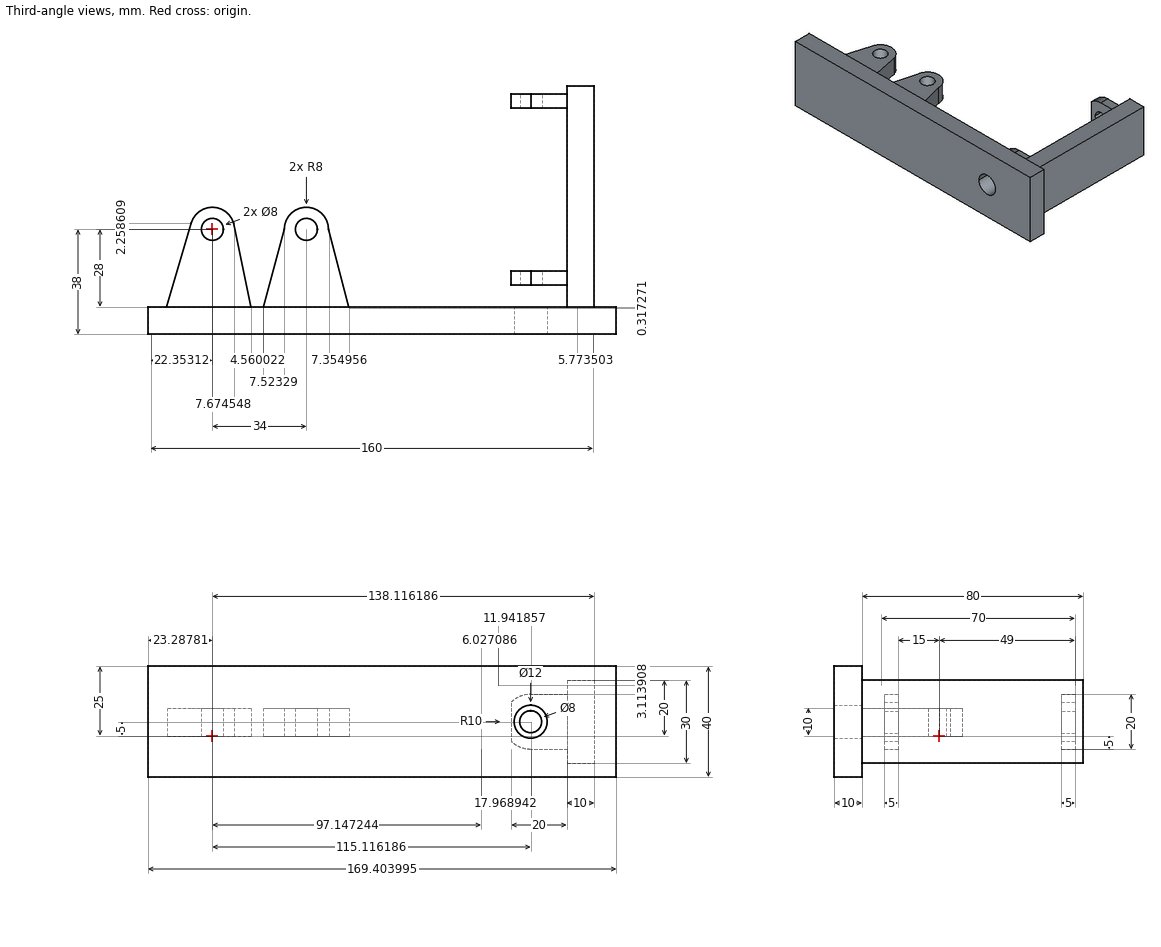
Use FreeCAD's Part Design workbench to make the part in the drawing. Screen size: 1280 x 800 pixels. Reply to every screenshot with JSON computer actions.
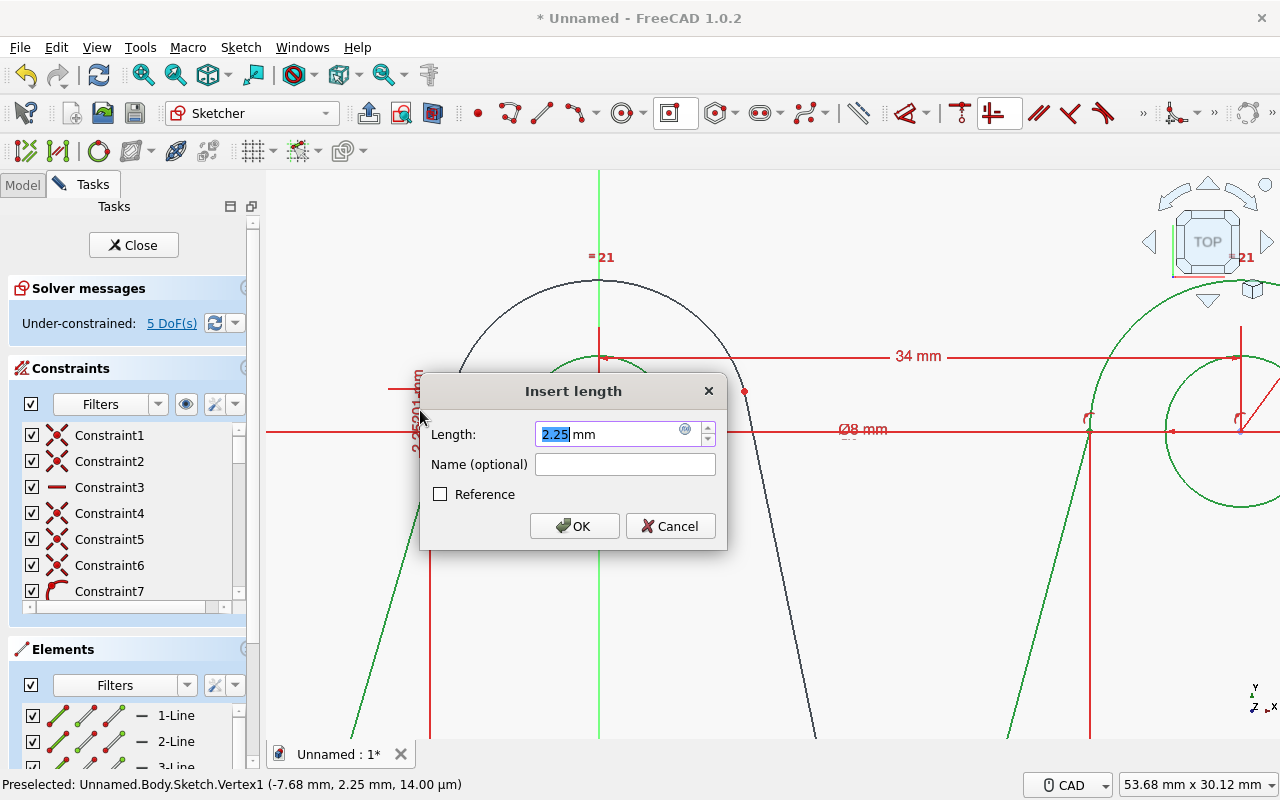
{"action": "type", "text": "2.258609"}
{"action": "key", "text": "Return"}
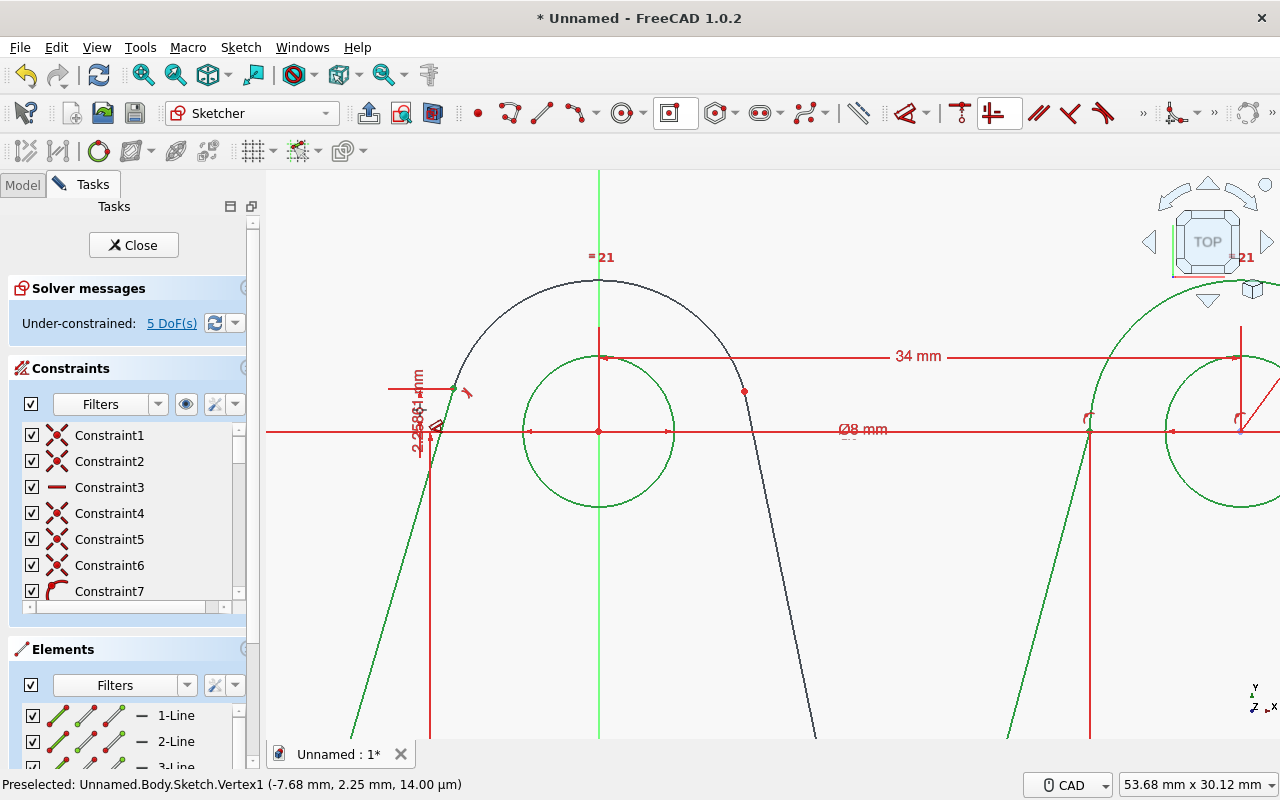
{"action": "scroll", "coordinate": [456, 389], "scroll_direction": "down", "scroll_amount": 8}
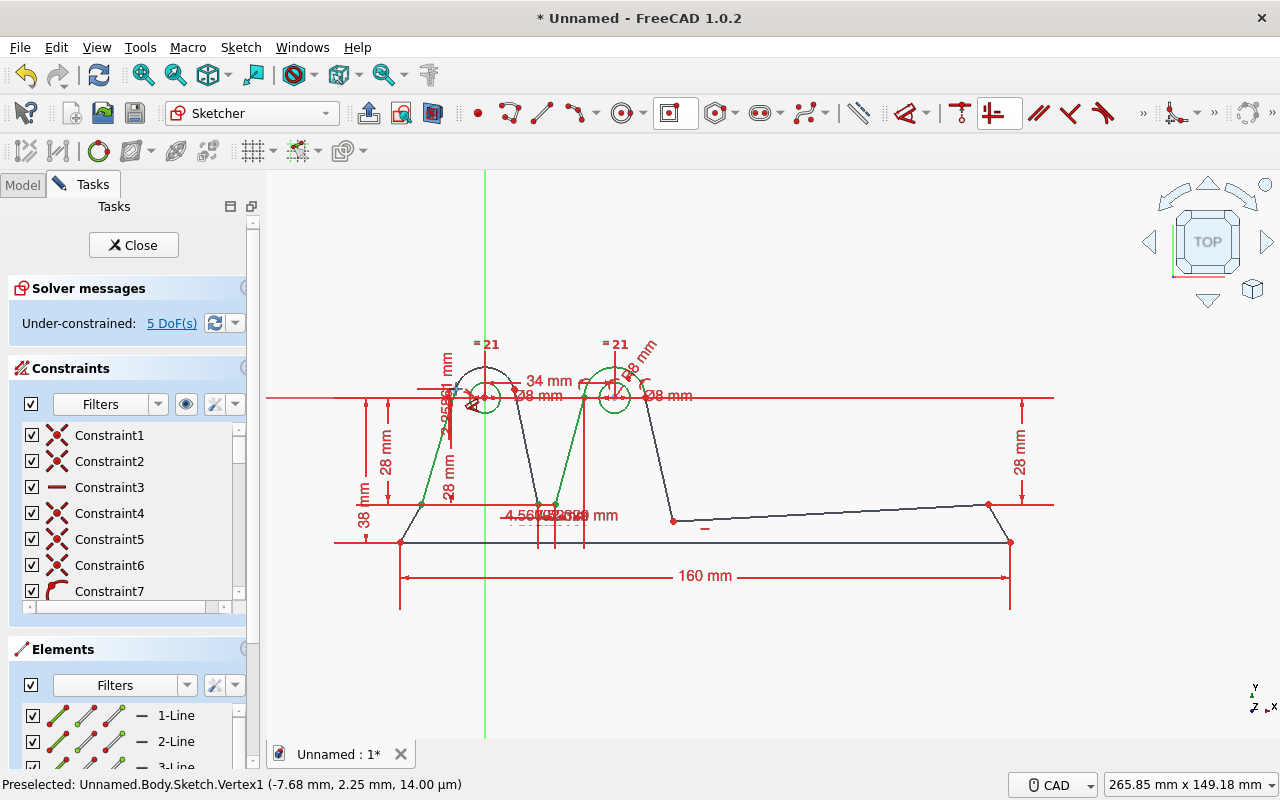
{"action": "left_click", "coordinate": [400, 543]}
{"action": "left_click", "coordinate": [442, 577]}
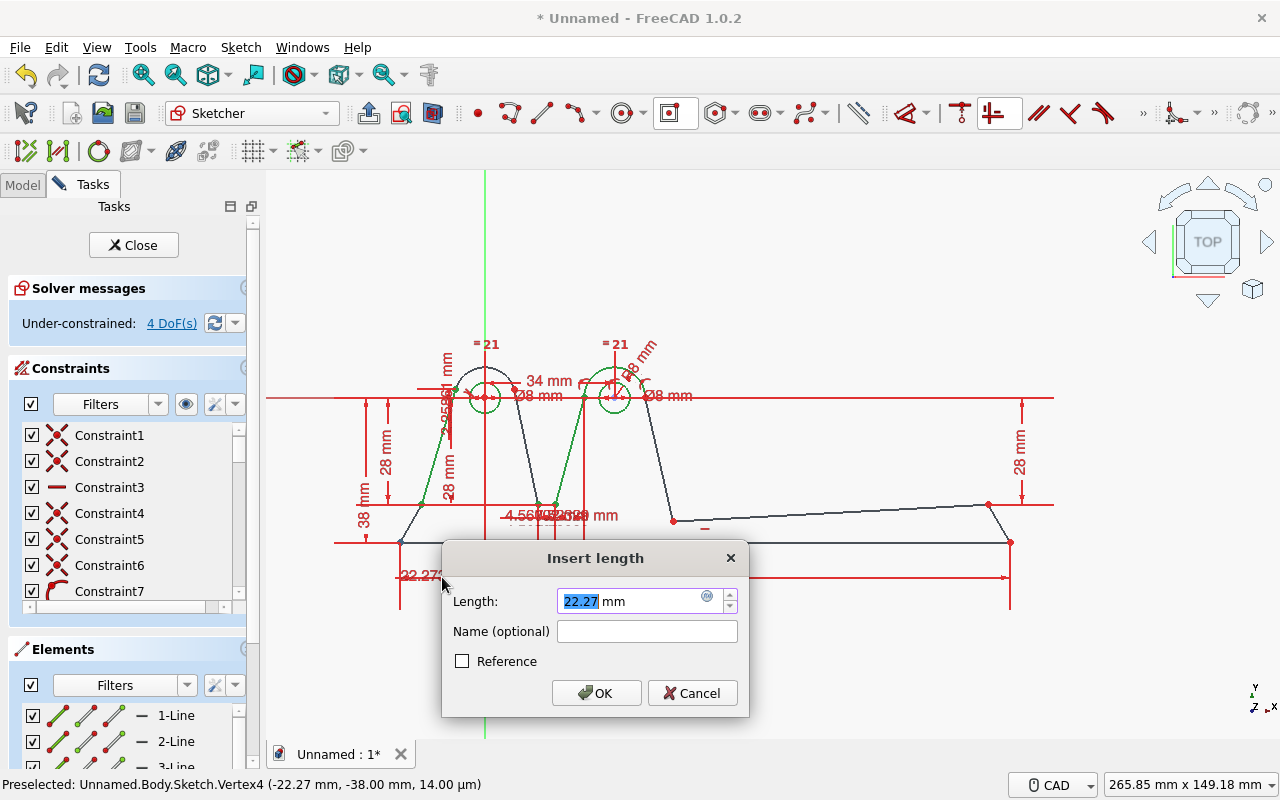
{"action": "type", "text": "22.35312"}
{"action": "key", "text": "Return"}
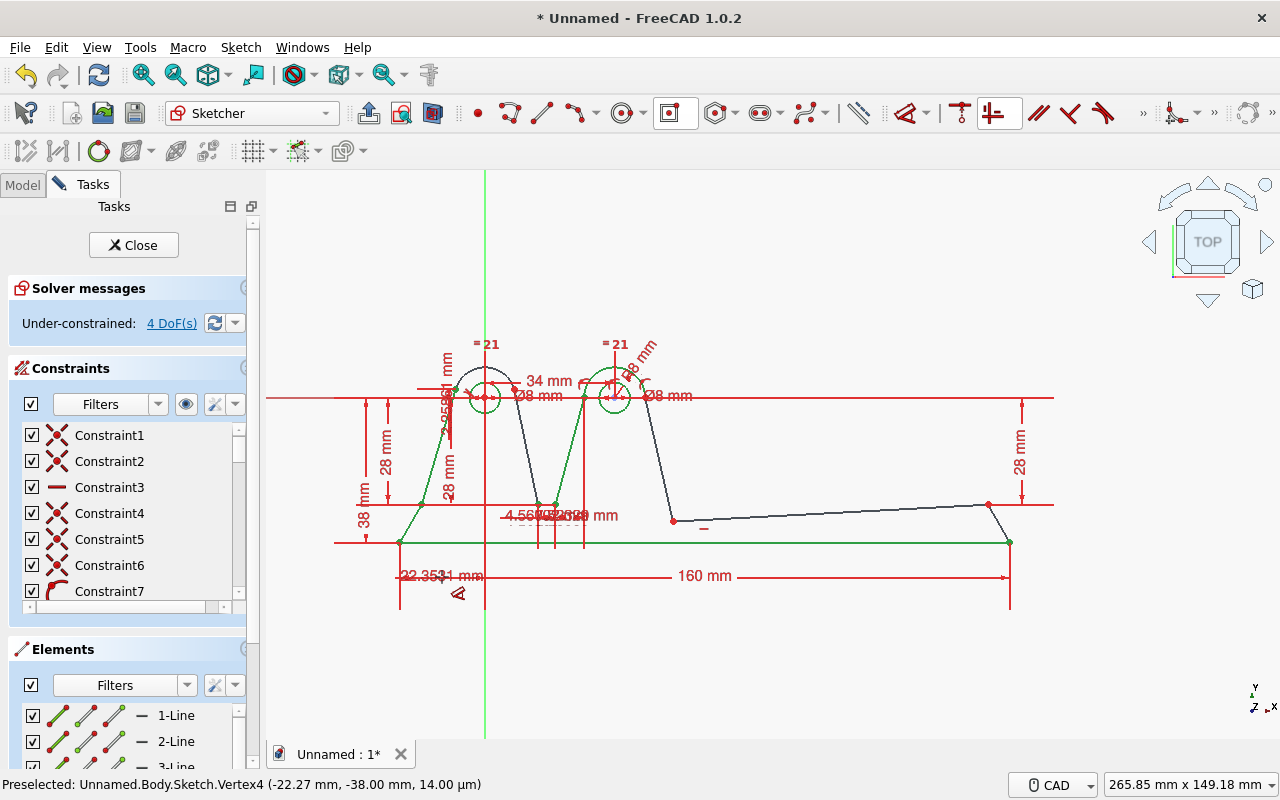
{"action": "scroll", "coordinate": [514, 390], "scroll_direction": "up", "scroll_amount": 2}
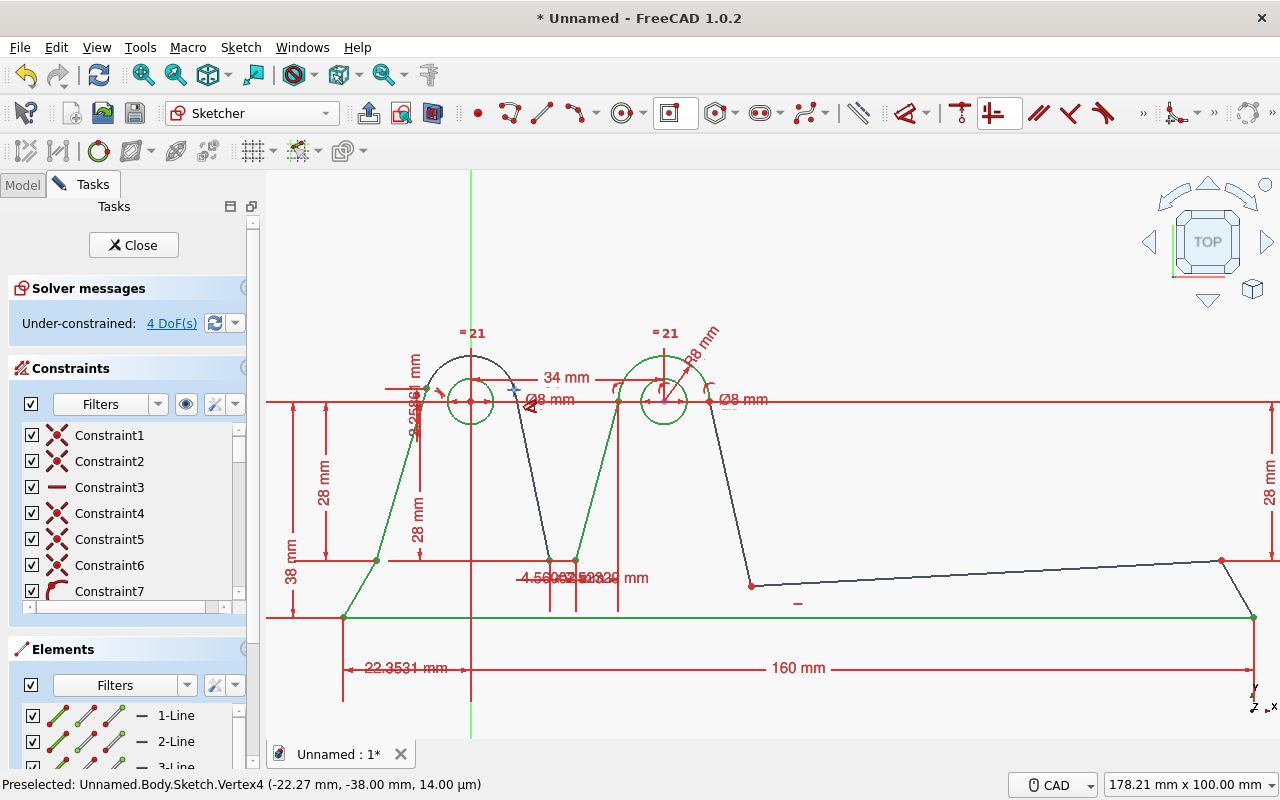
{"action": "left_click", "coordinate": [514, 390]}
{"action": "left_click", "coordinate": [508, 356]}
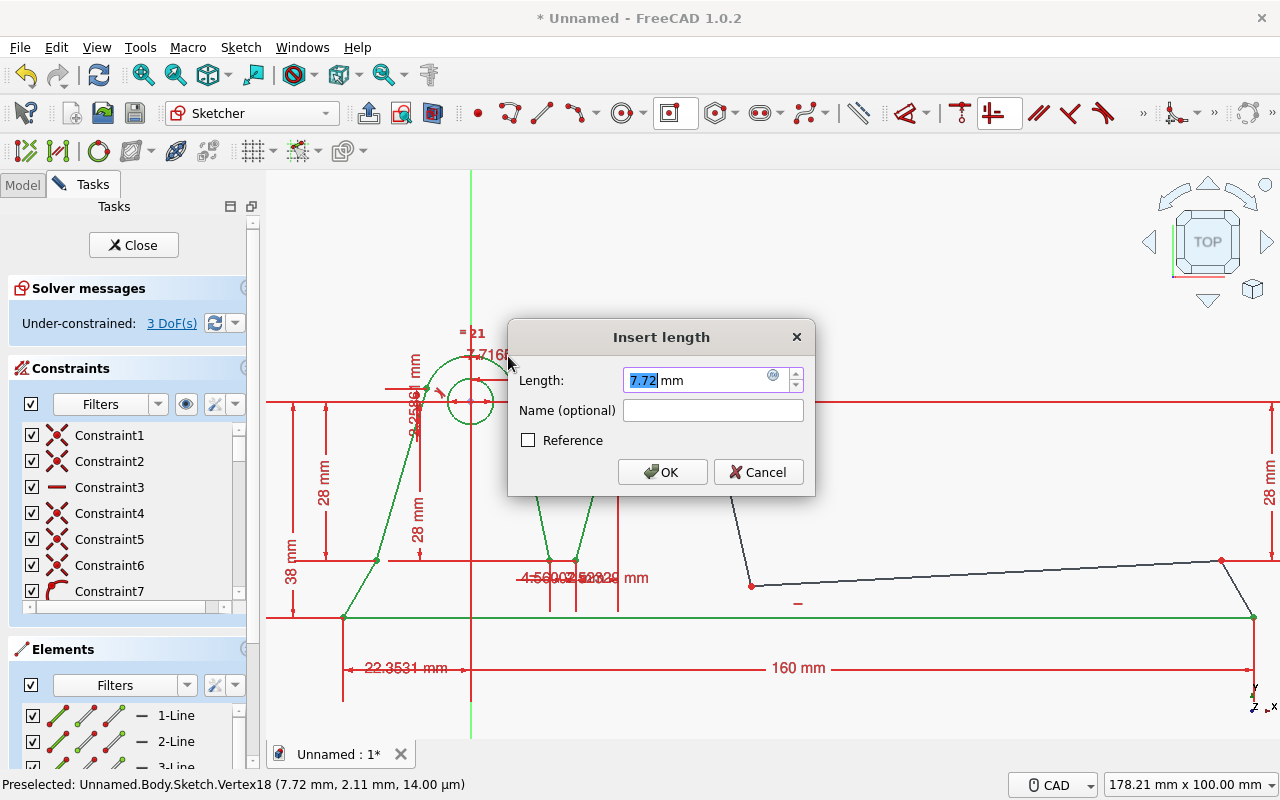
{"action": "type", "text": "7.674548"}
{"action": "key", "text": "Return"}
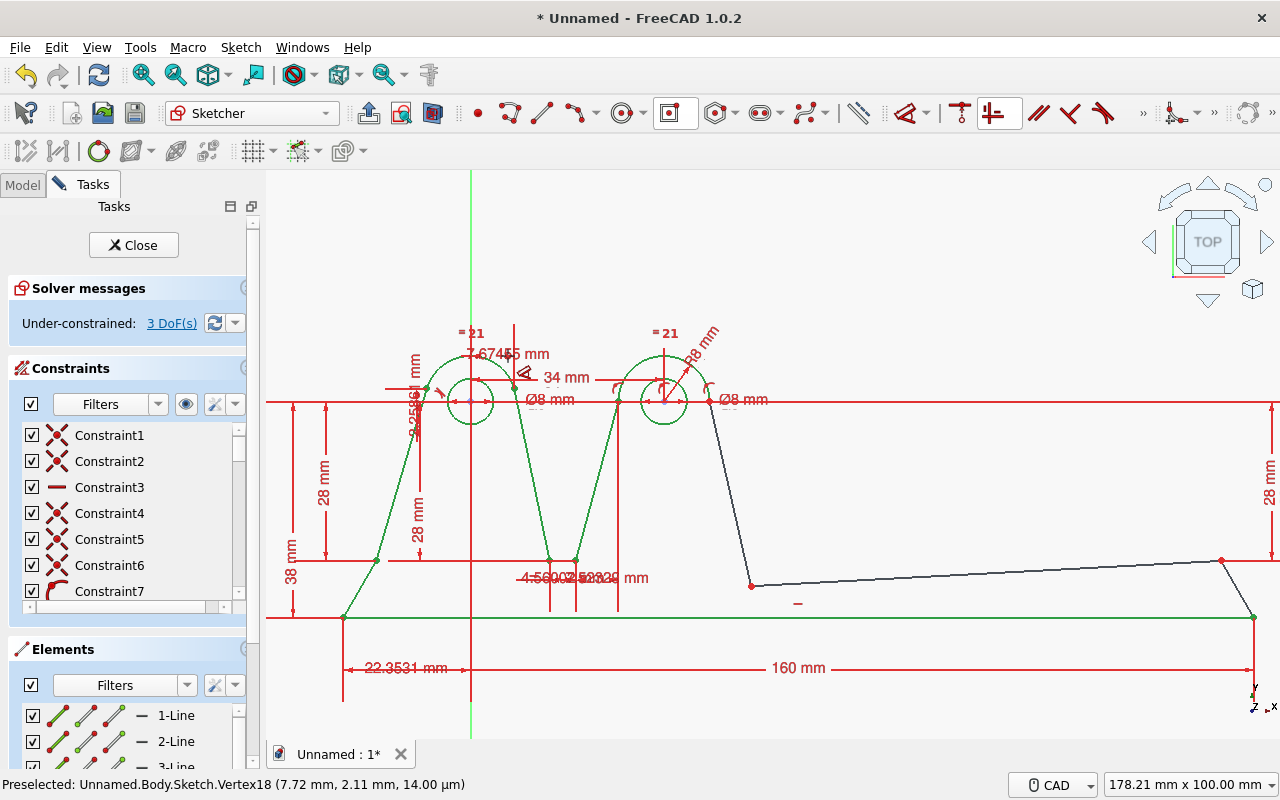
{"action": "scroll", "coordinate": [513, 389], "scroll_direction": "down", "scroll_amount": 2}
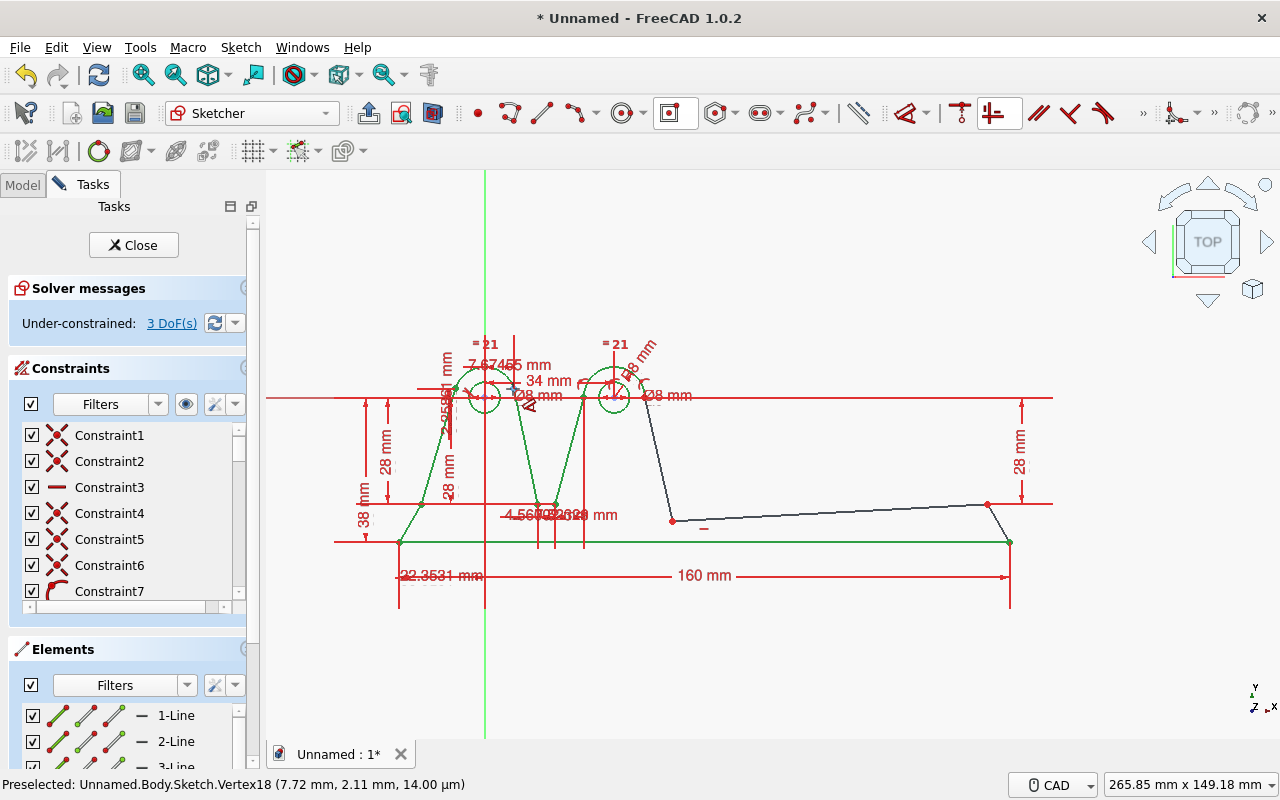
{"action": "scroll", "coordinate": [1003, 531], "scroll_direction": "up", "scroll_amount": 3}